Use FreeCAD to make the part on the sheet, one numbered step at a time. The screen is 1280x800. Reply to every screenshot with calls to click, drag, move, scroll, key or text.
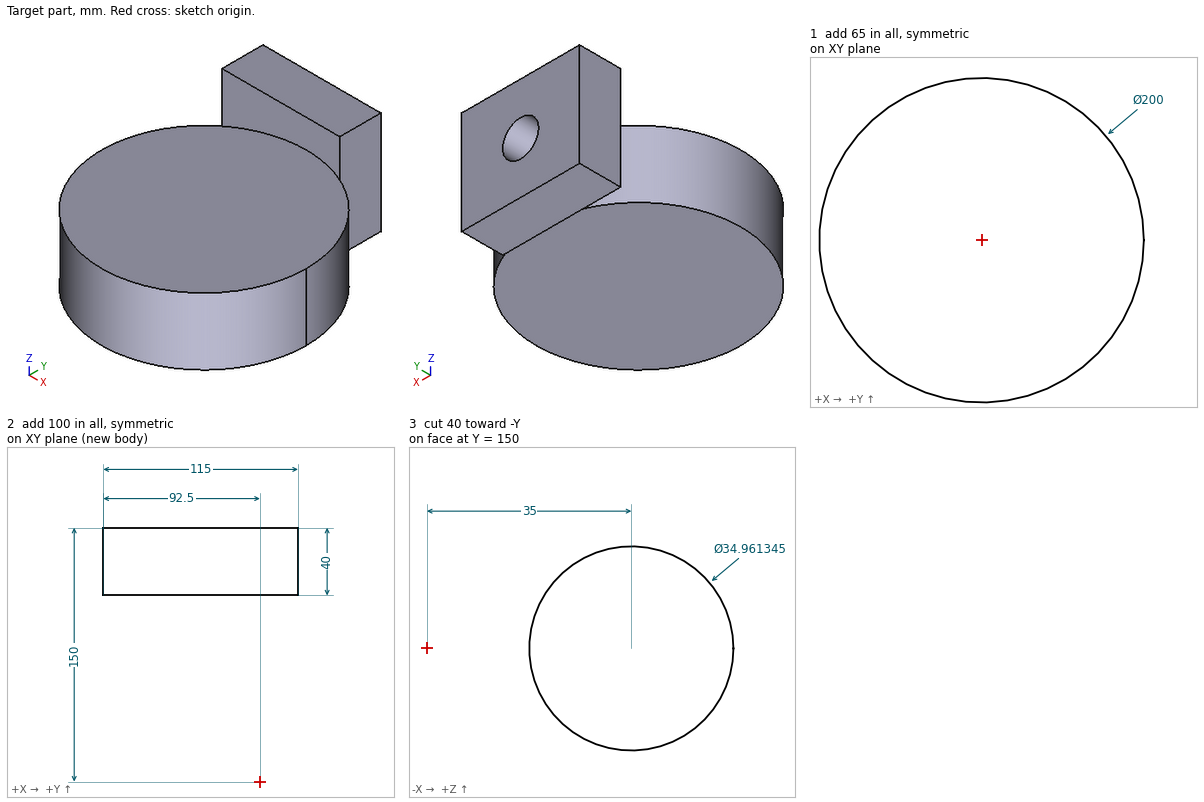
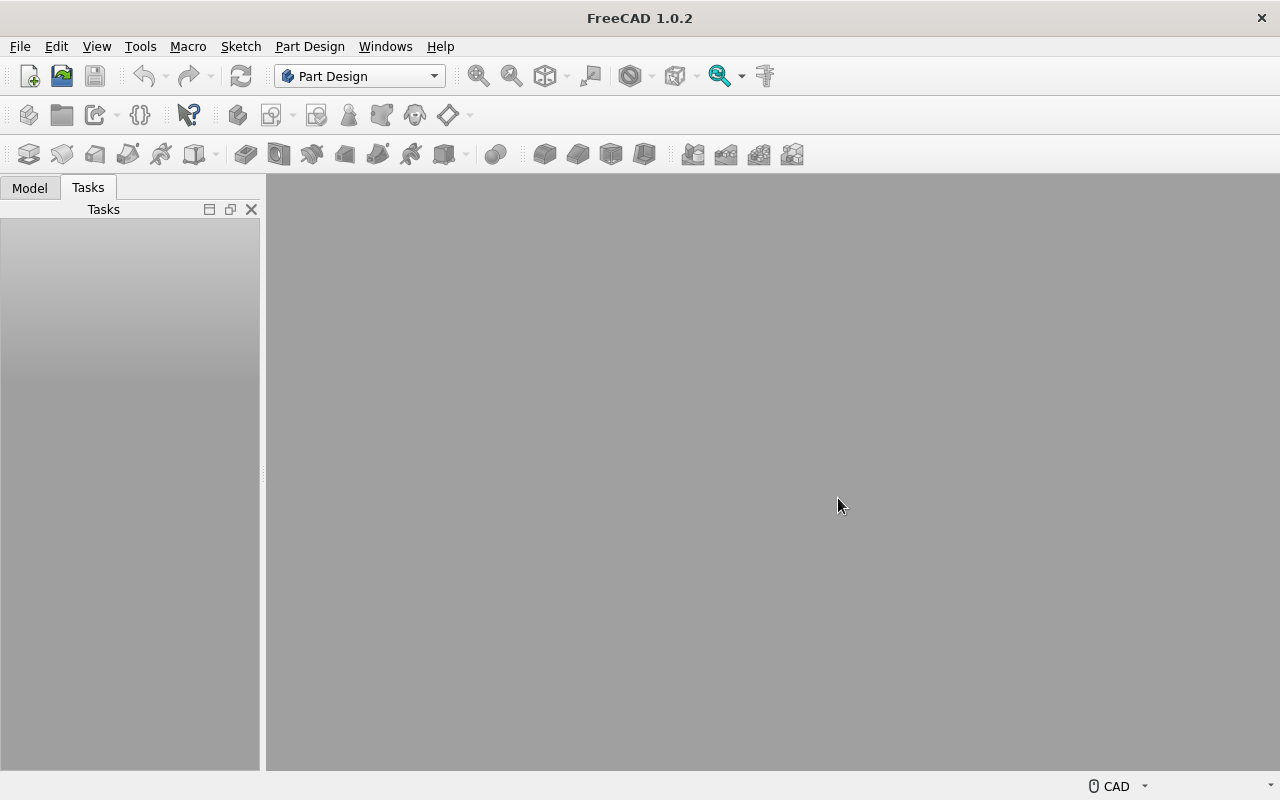
key(ctrl+n)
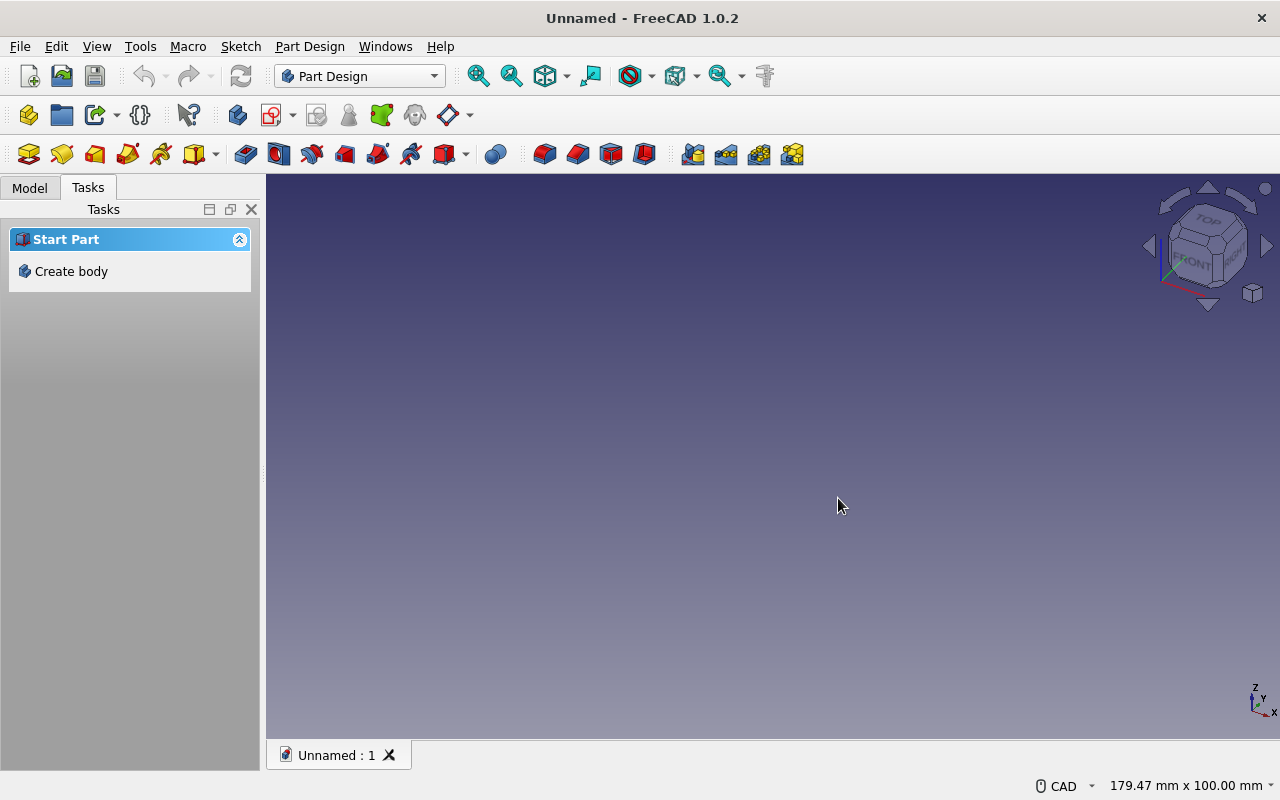
click(270, 116)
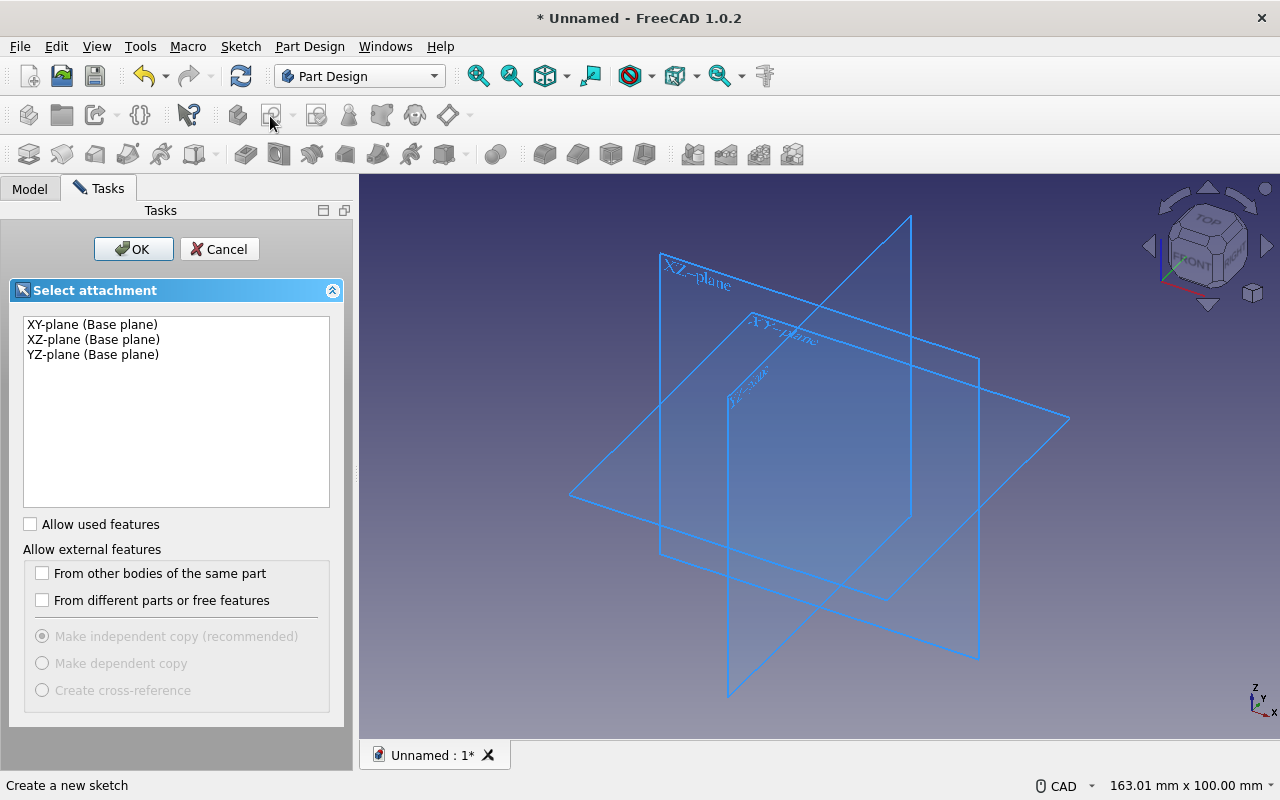
click(84, 324)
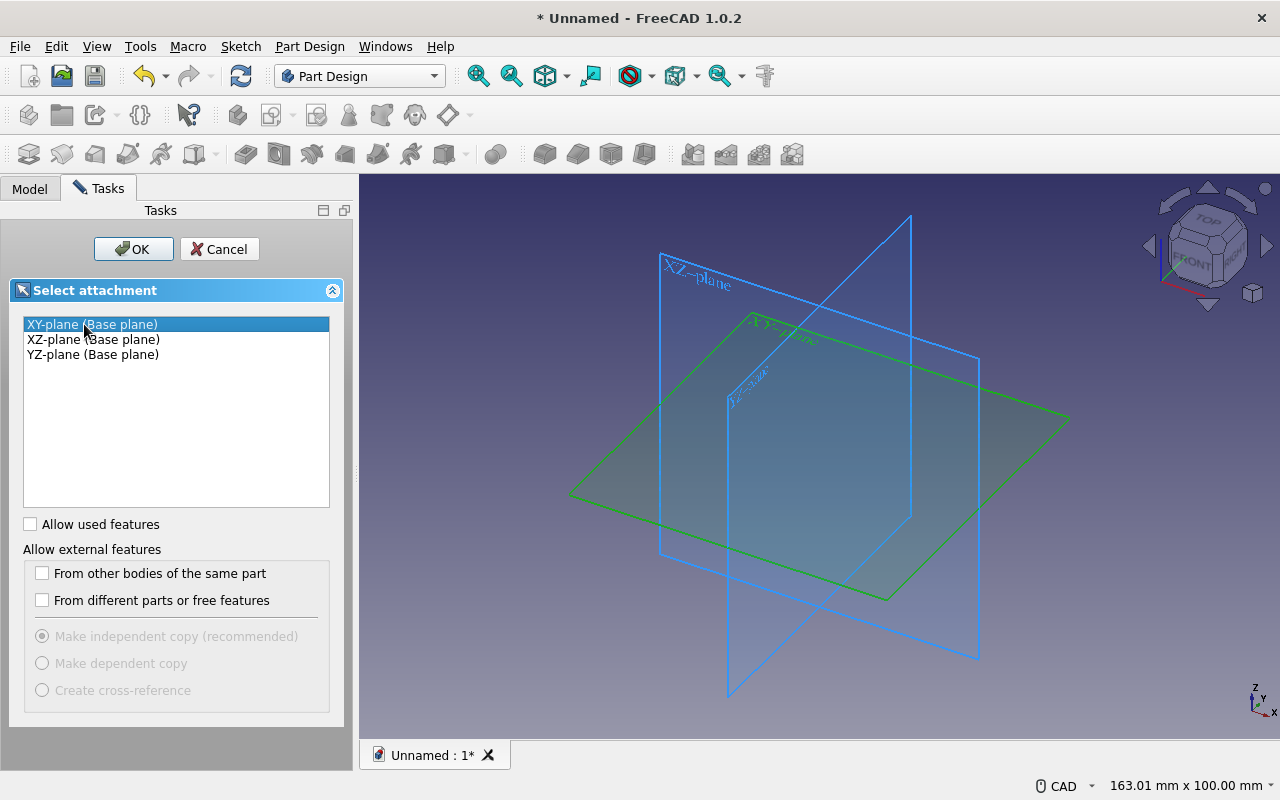
click(134, 249)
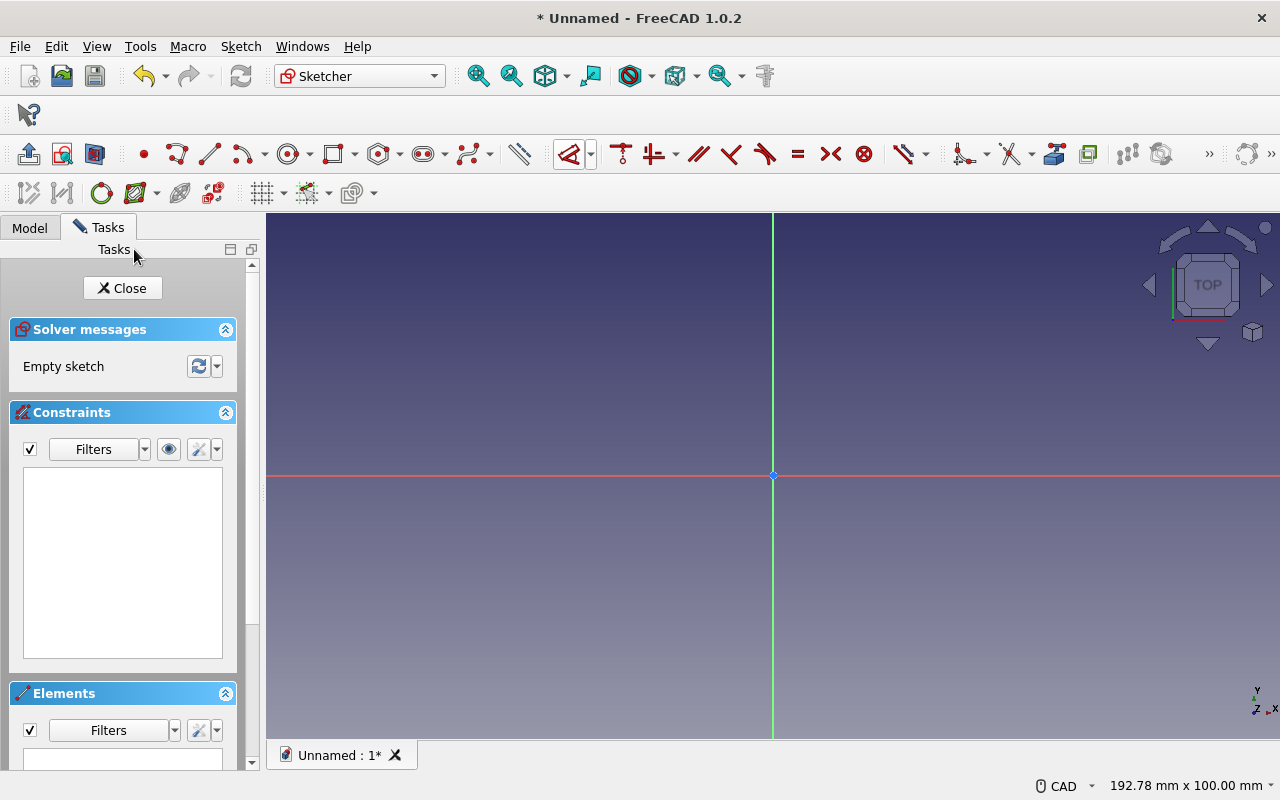
scroll(675, 476, down, 6)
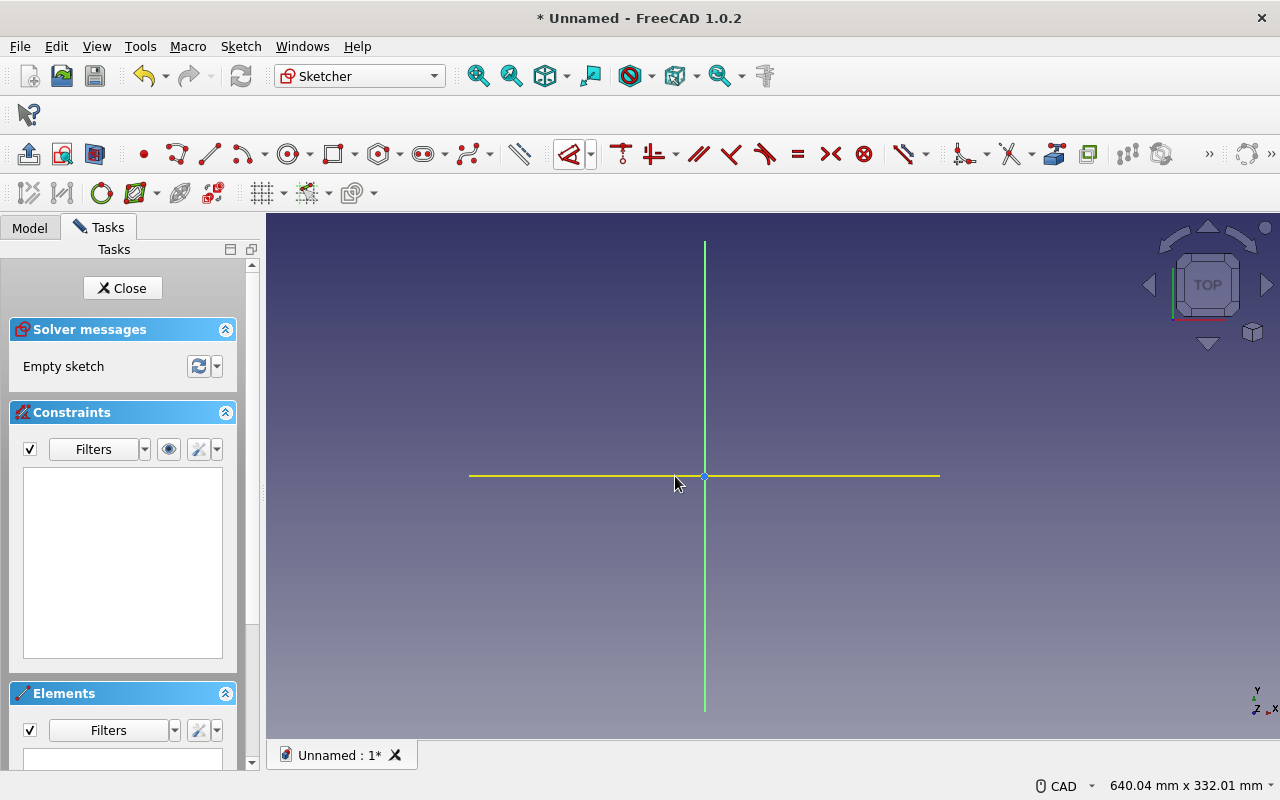
click(288, 154)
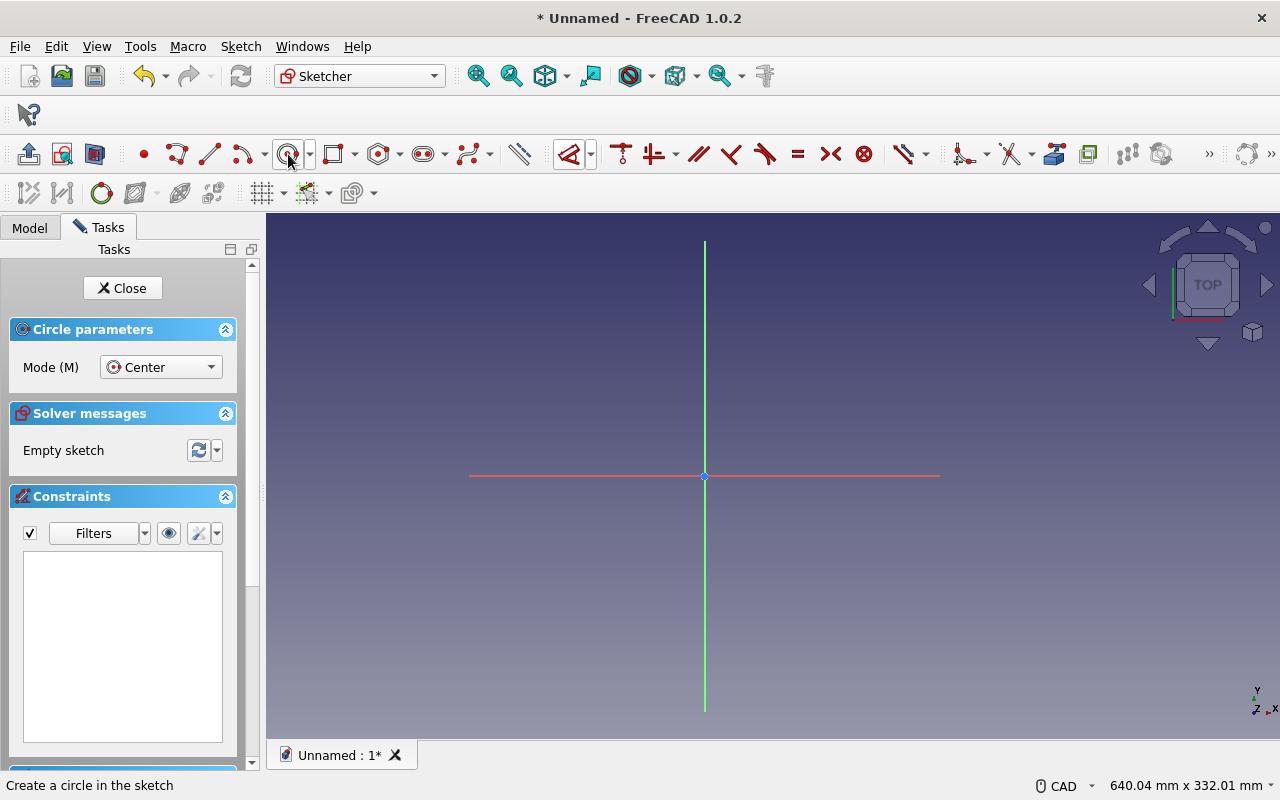
click(705, 476)
move(817, 364)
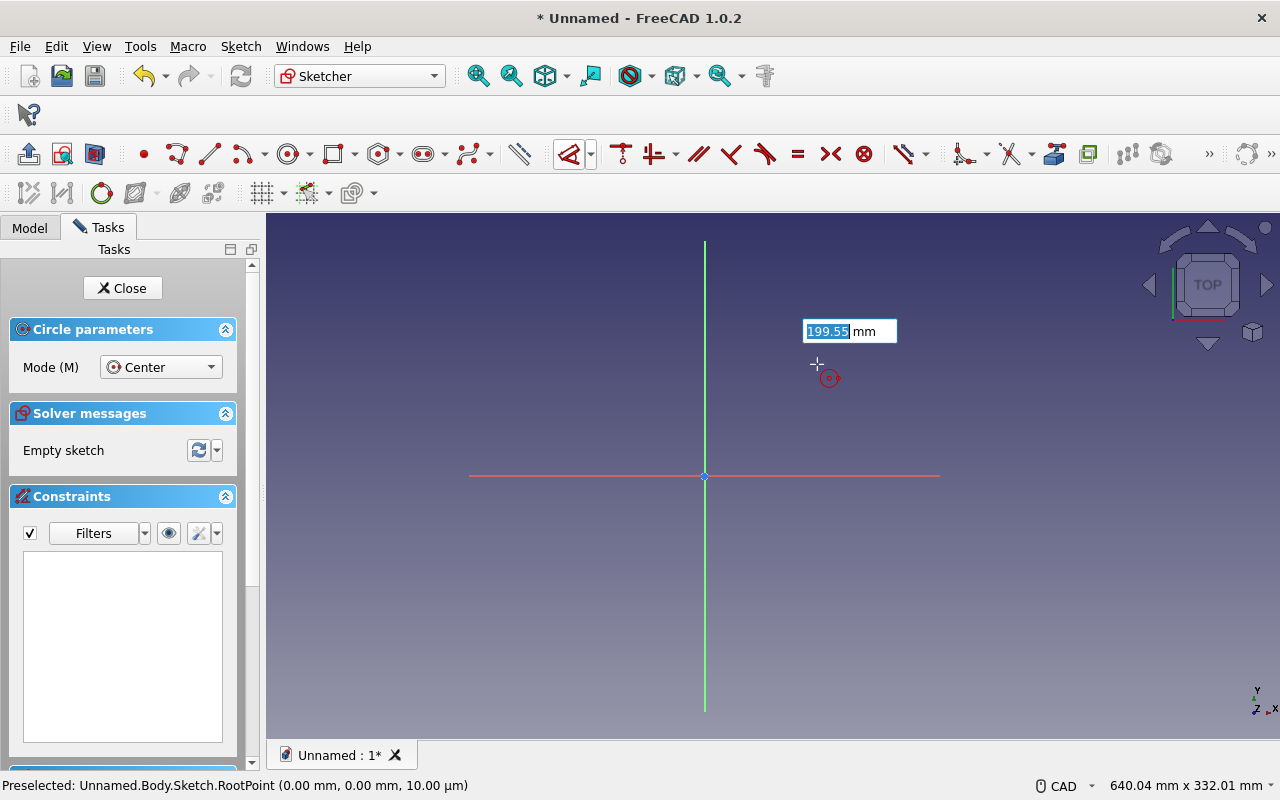
text(200)
key(Return)
key(Escape)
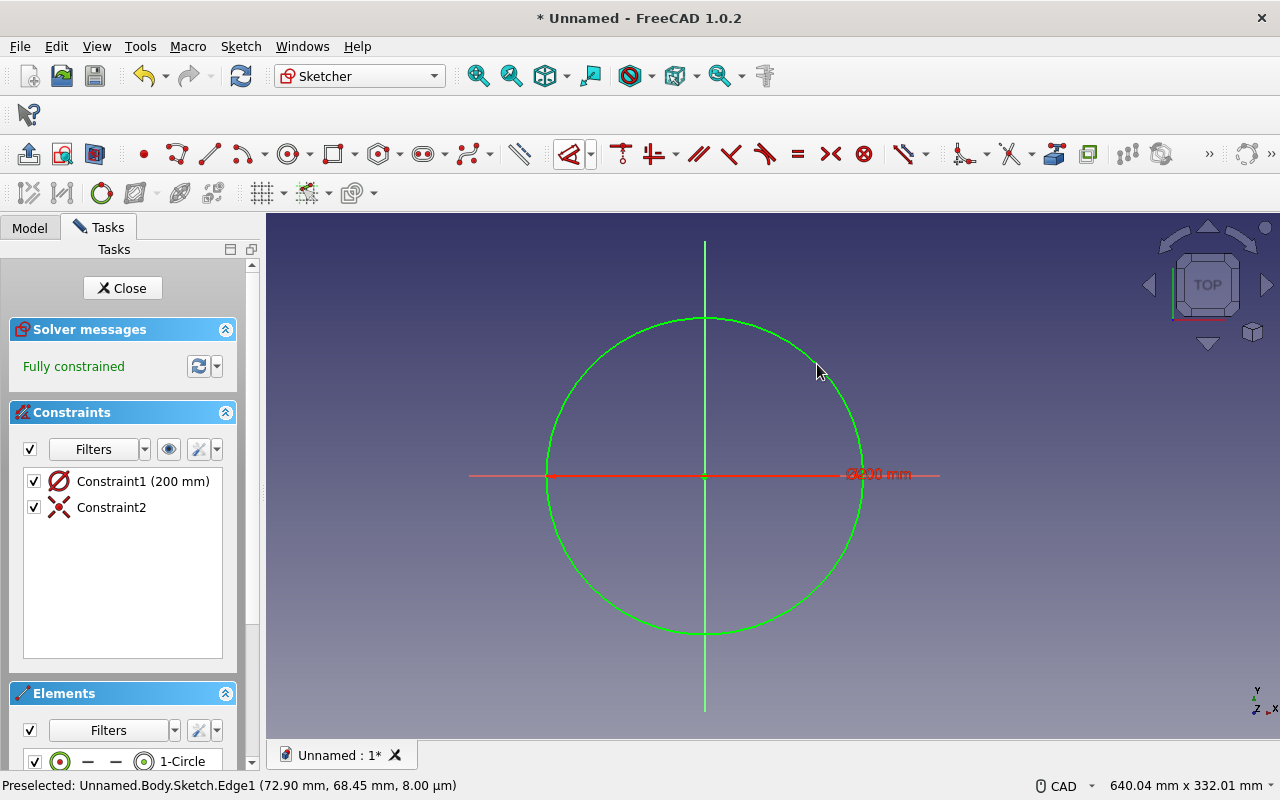
click(123, 288)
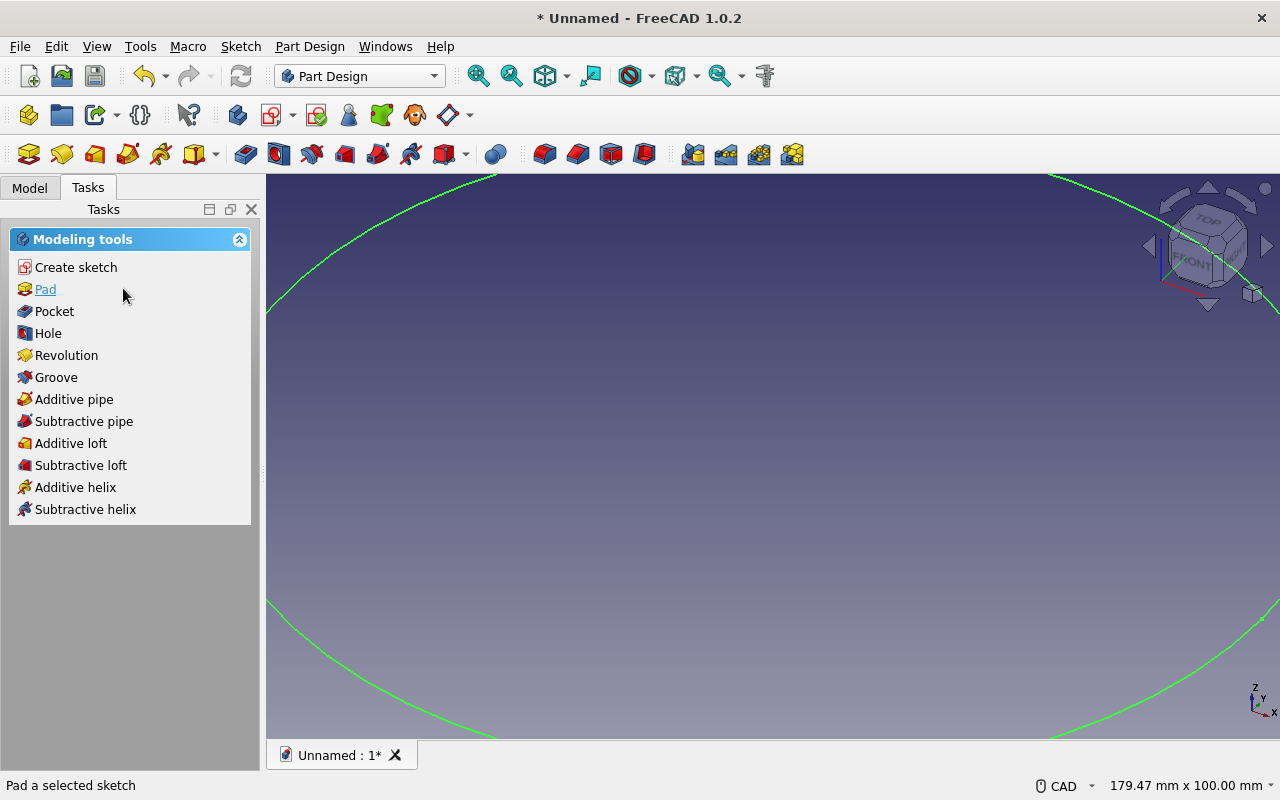
click(29, 154)